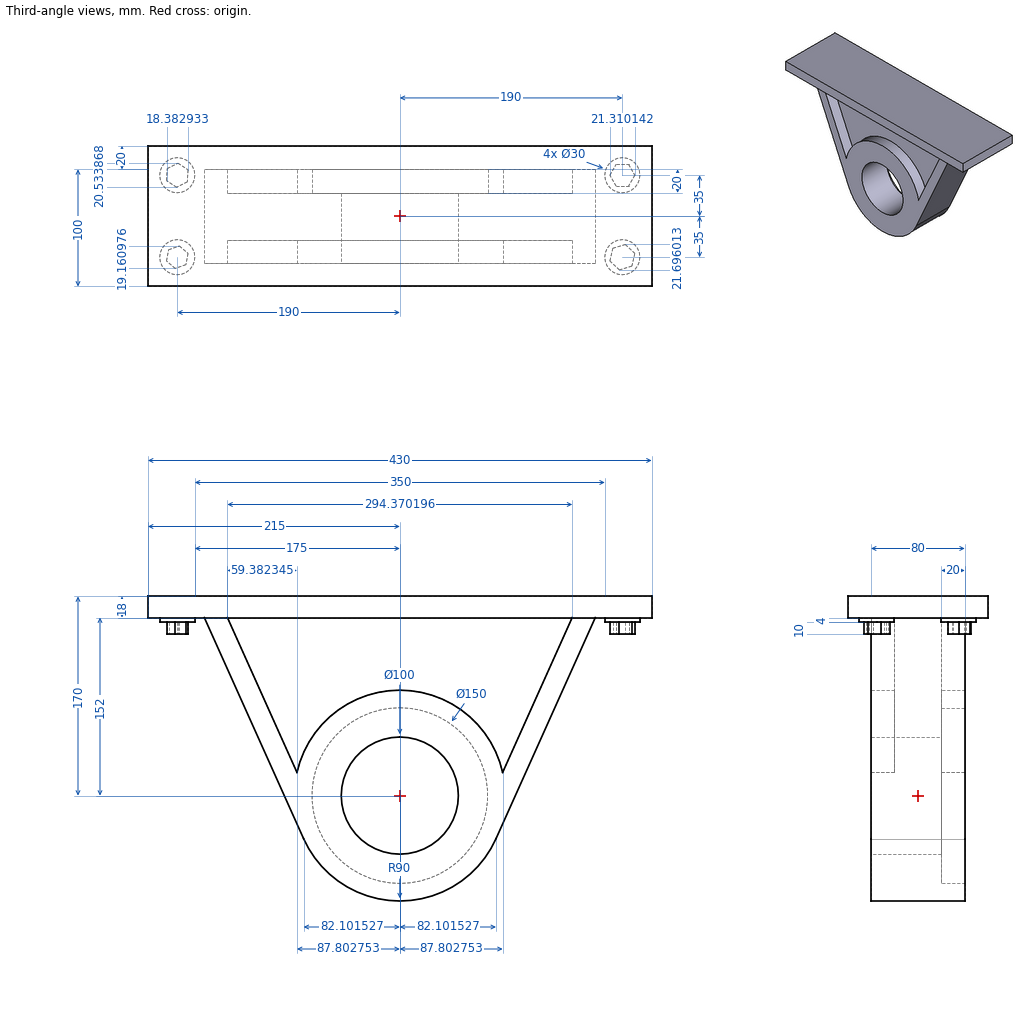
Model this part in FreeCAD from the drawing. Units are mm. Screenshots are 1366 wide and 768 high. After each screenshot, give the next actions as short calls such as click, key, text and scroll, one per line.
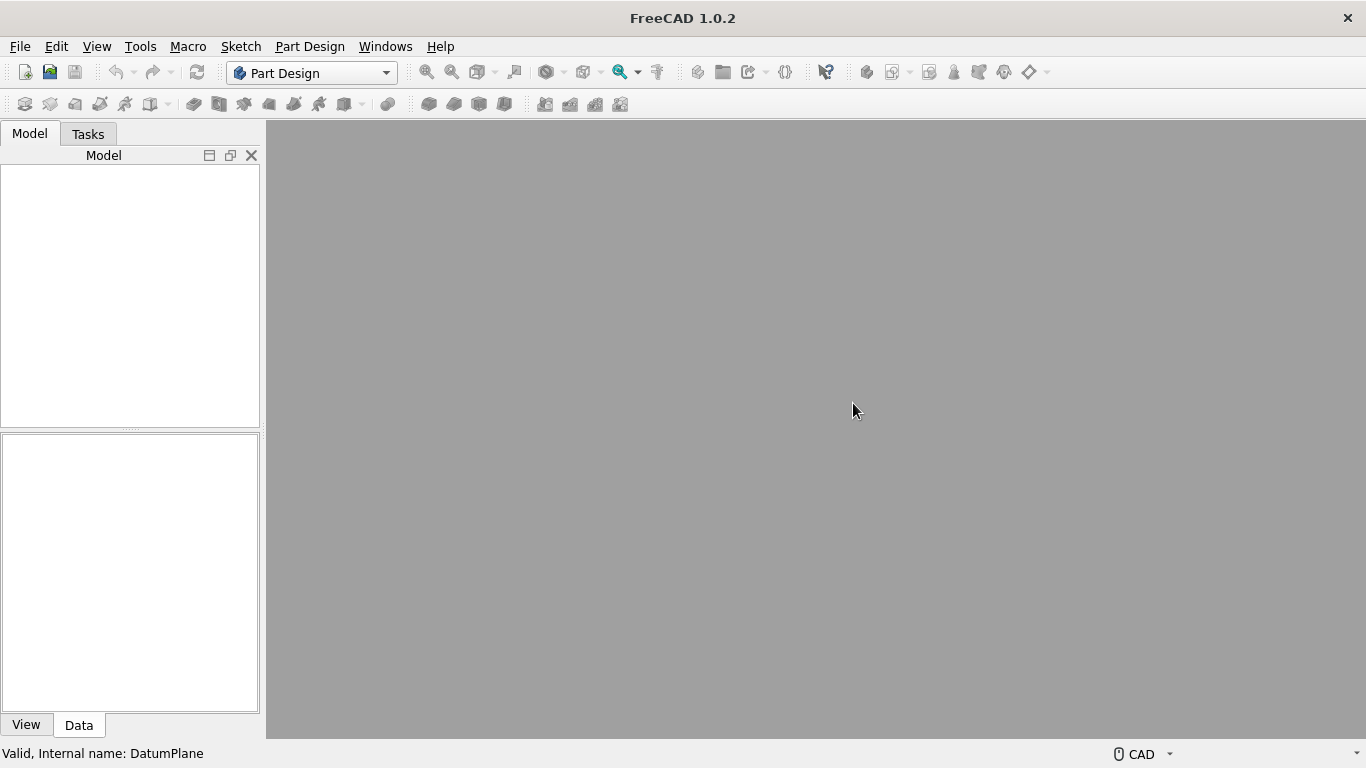
click(25, 72)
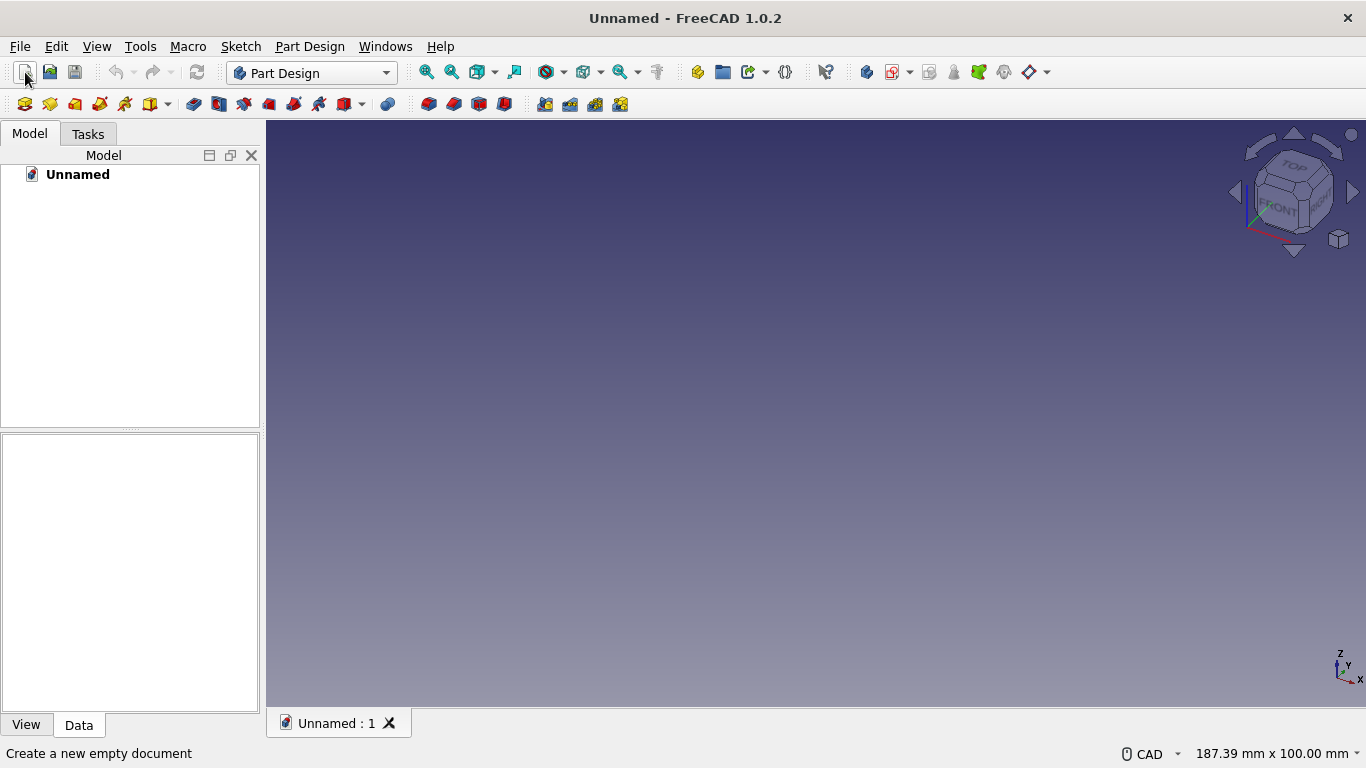
click(892, 72)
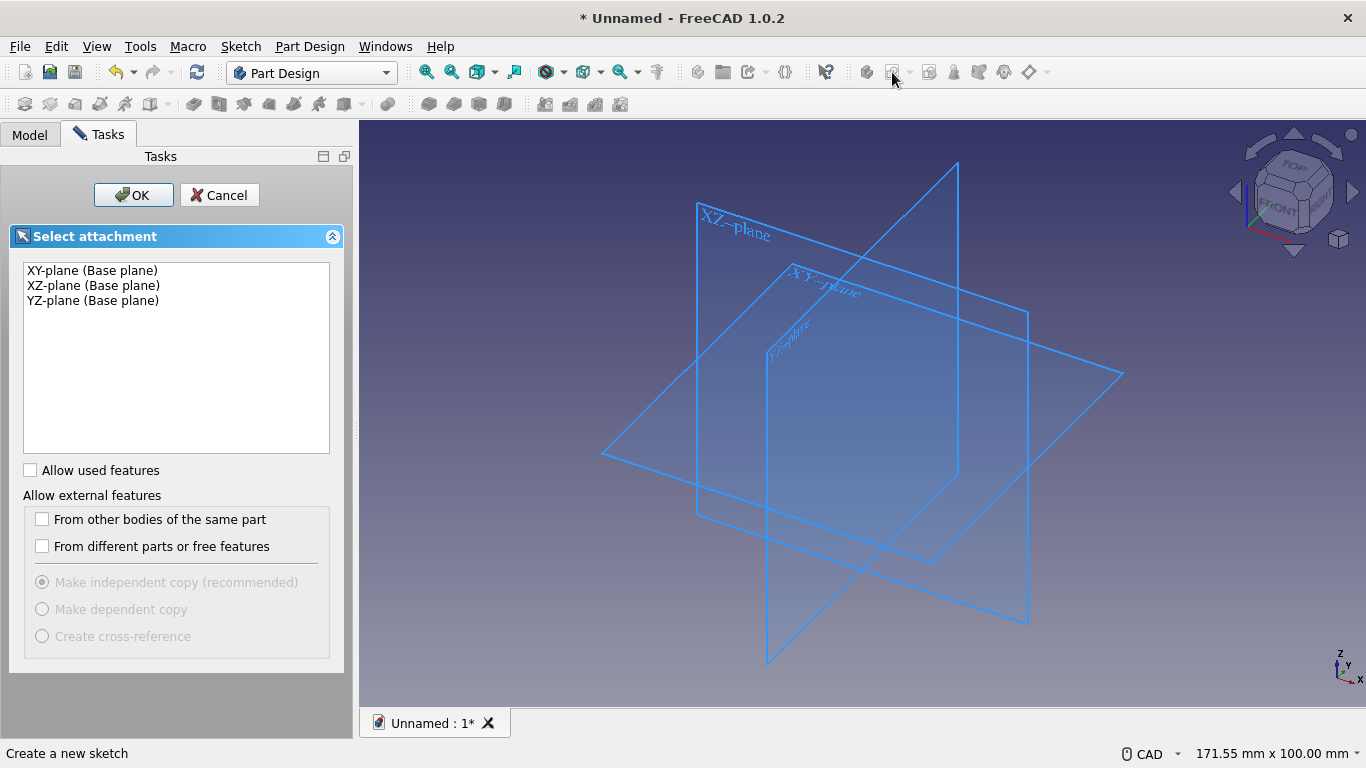
click(84, 286)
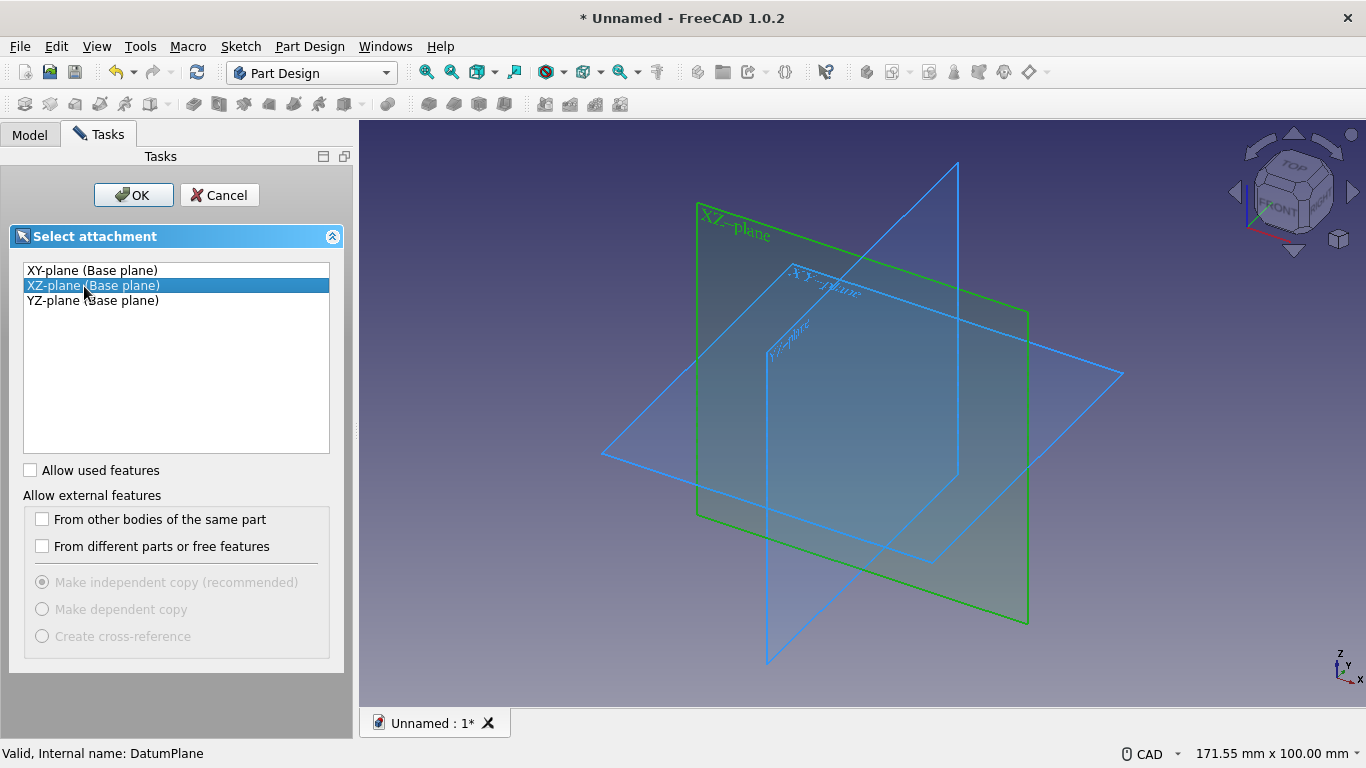
click(134, 195)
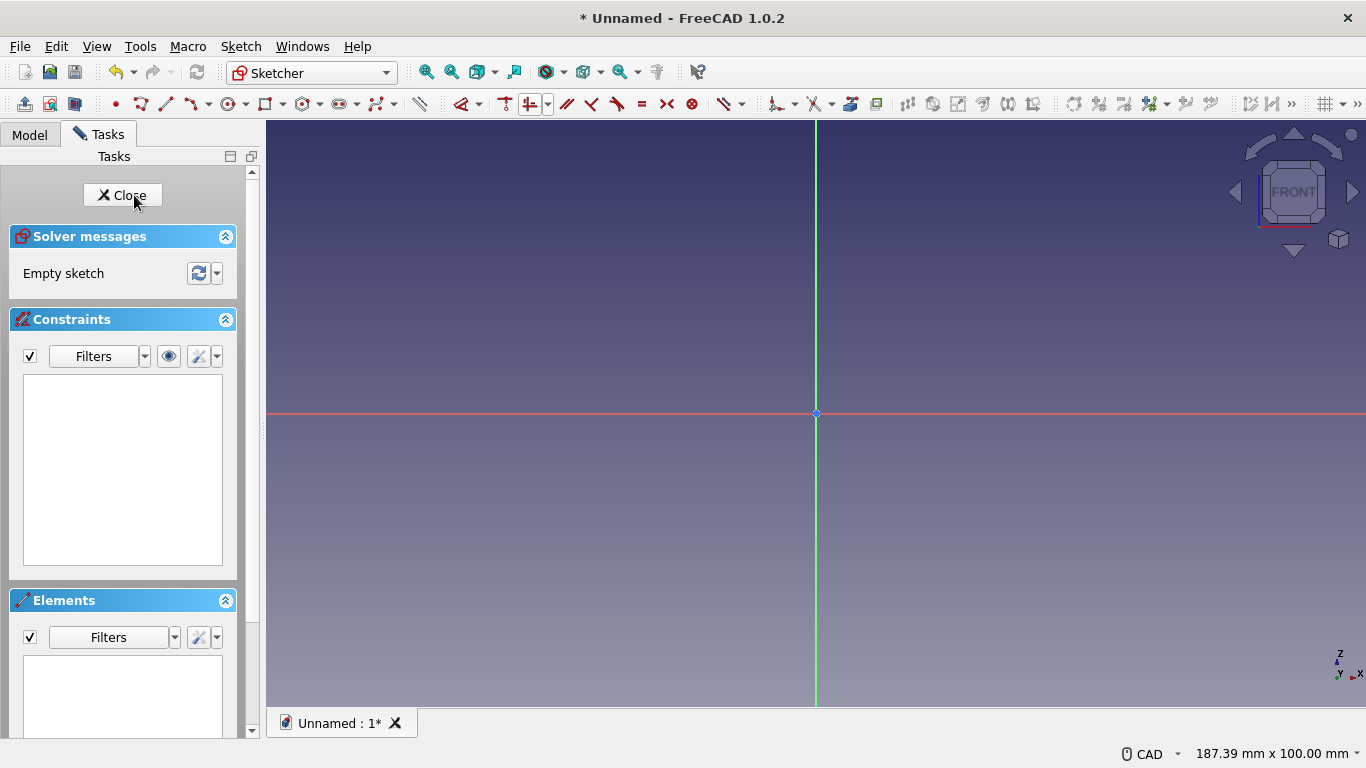
scroll(725, 490, down, 7)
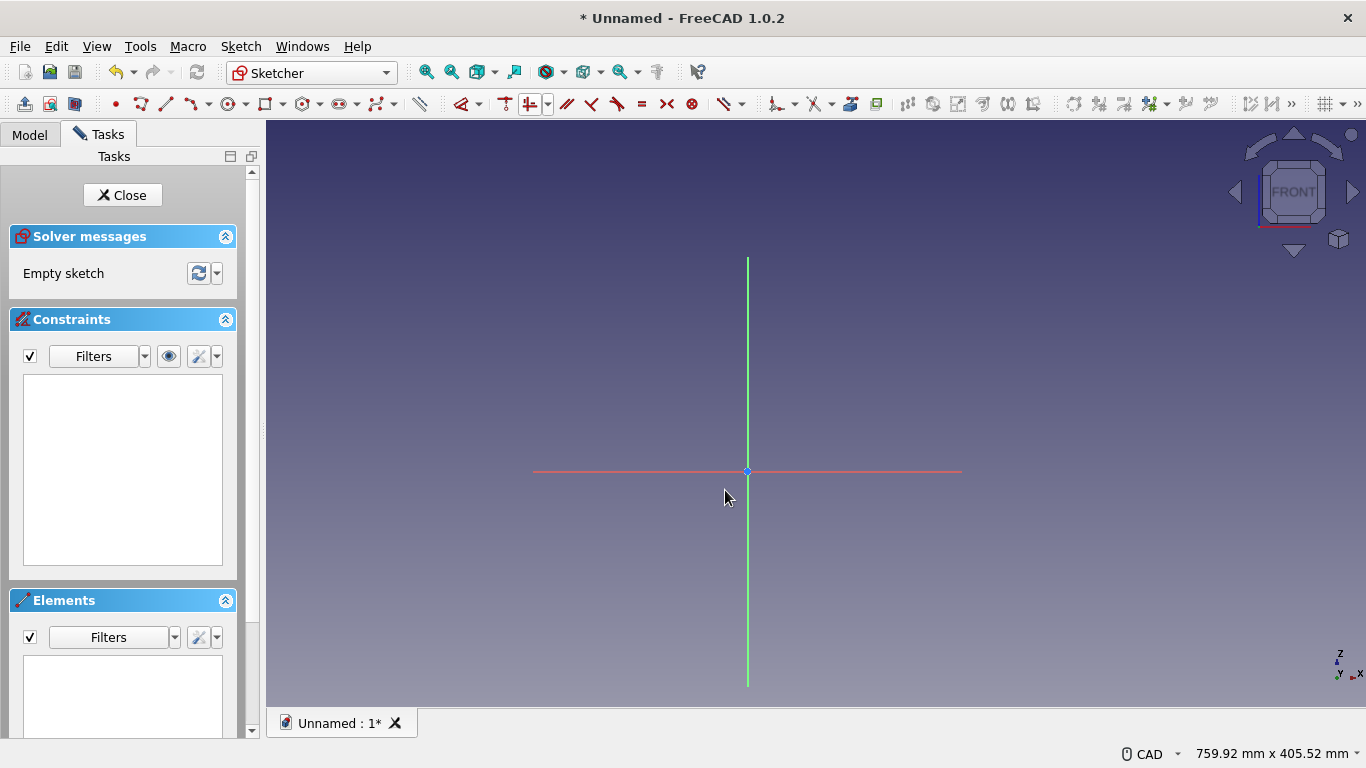
click(141, 104)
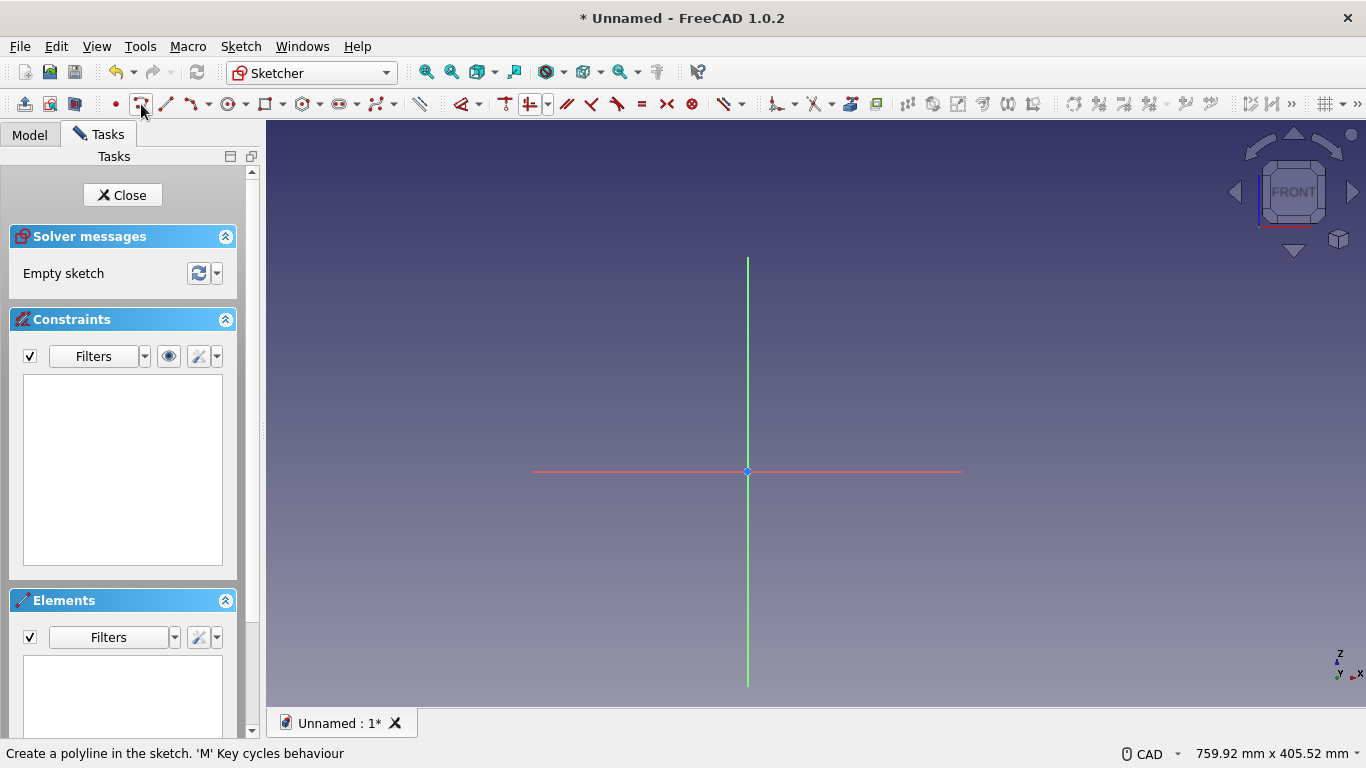
click(629, 525)
click(494, 226)
click(1001, 226)
click(867, 525)
right_click(867, 525)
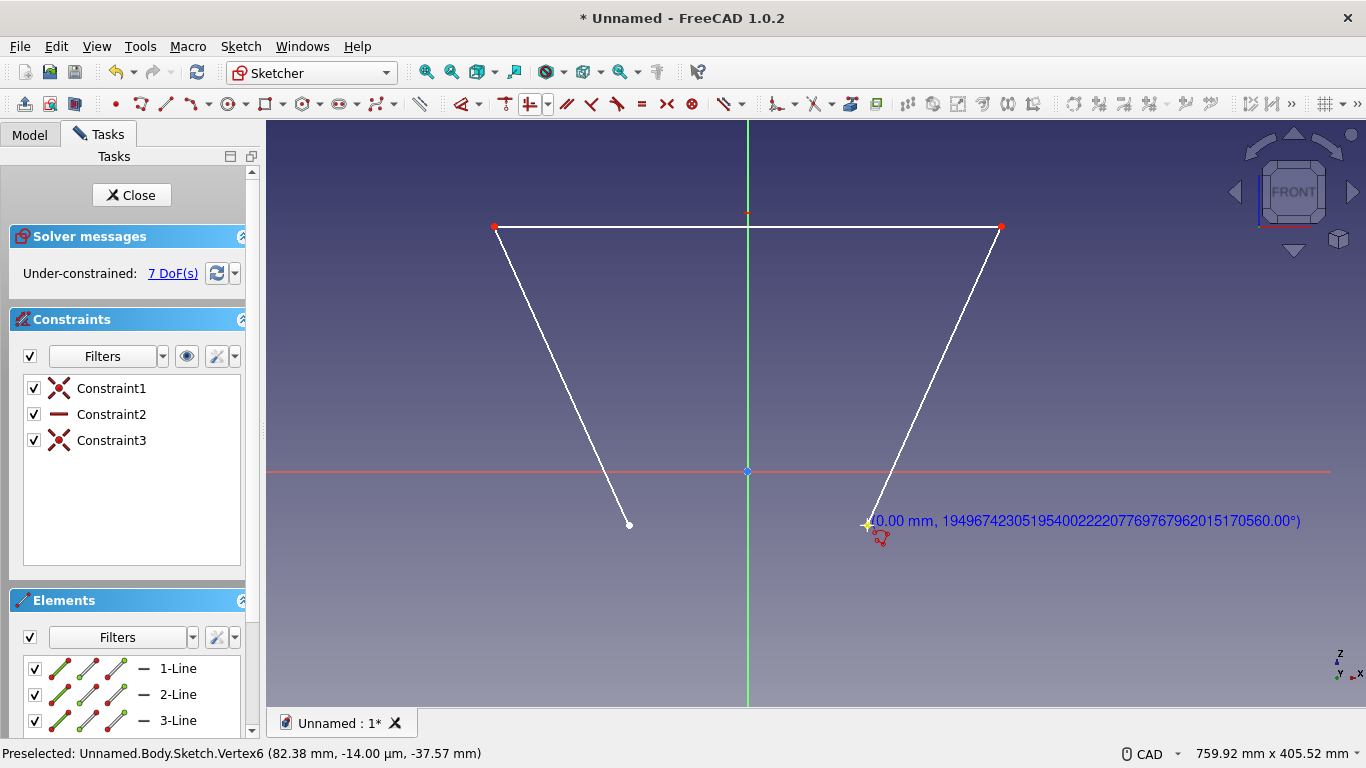
click(190, 104)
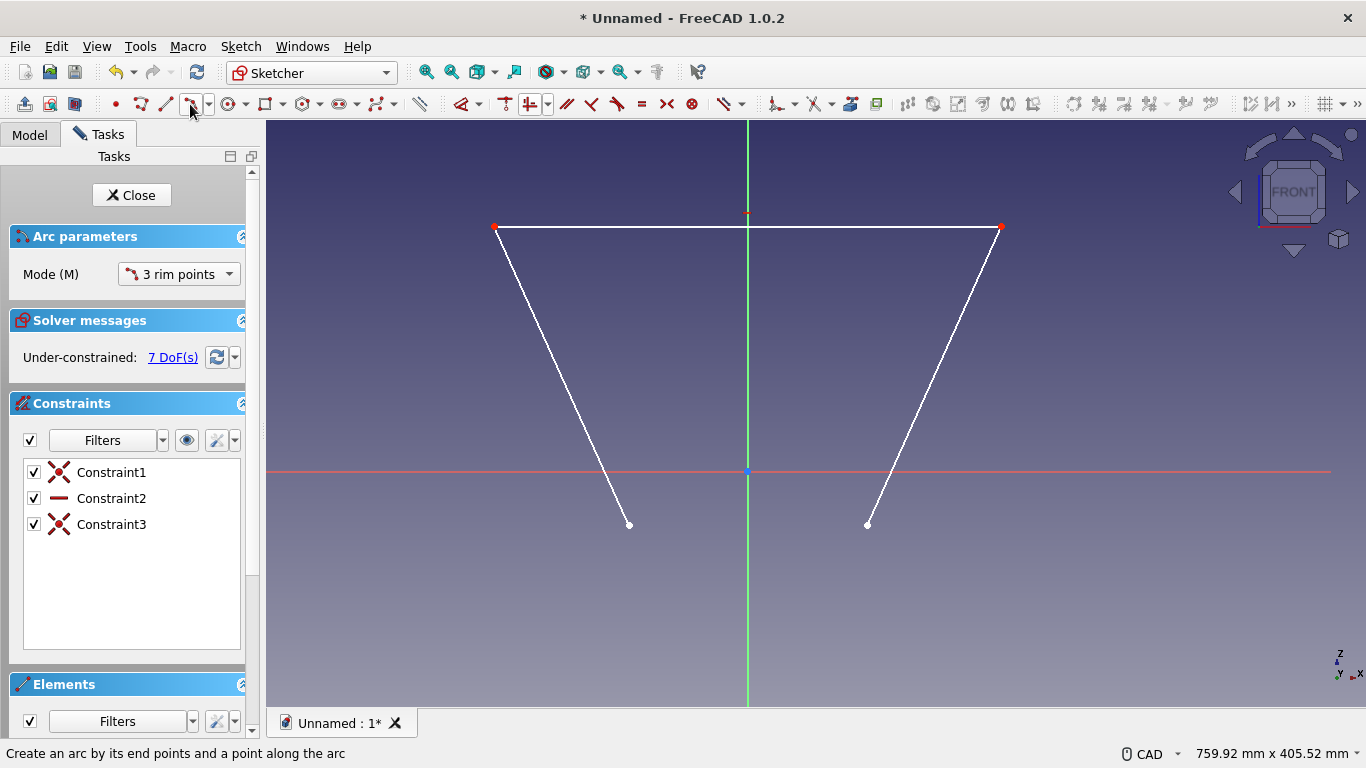
click(867, 526)
click(629, 526)
click(718, 598)